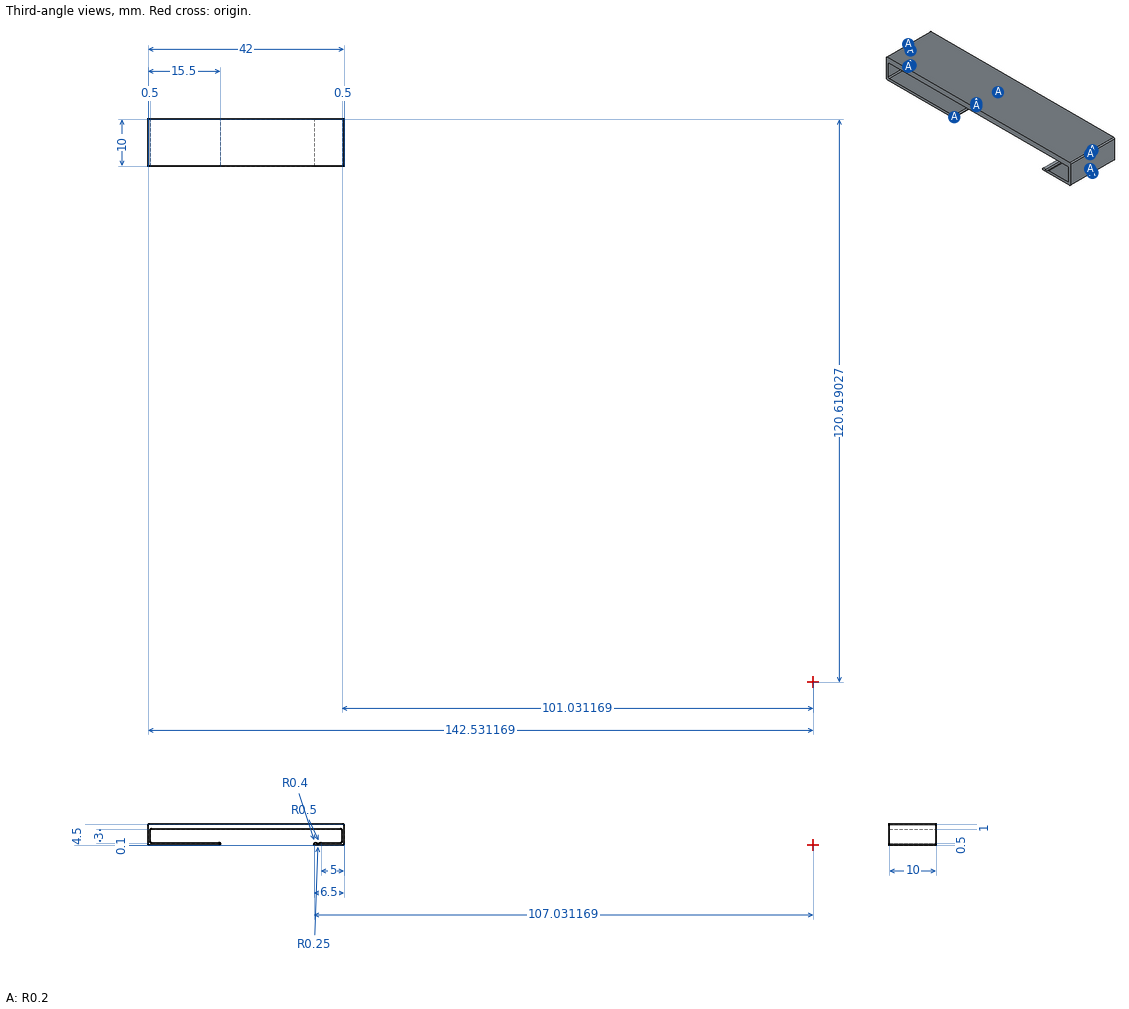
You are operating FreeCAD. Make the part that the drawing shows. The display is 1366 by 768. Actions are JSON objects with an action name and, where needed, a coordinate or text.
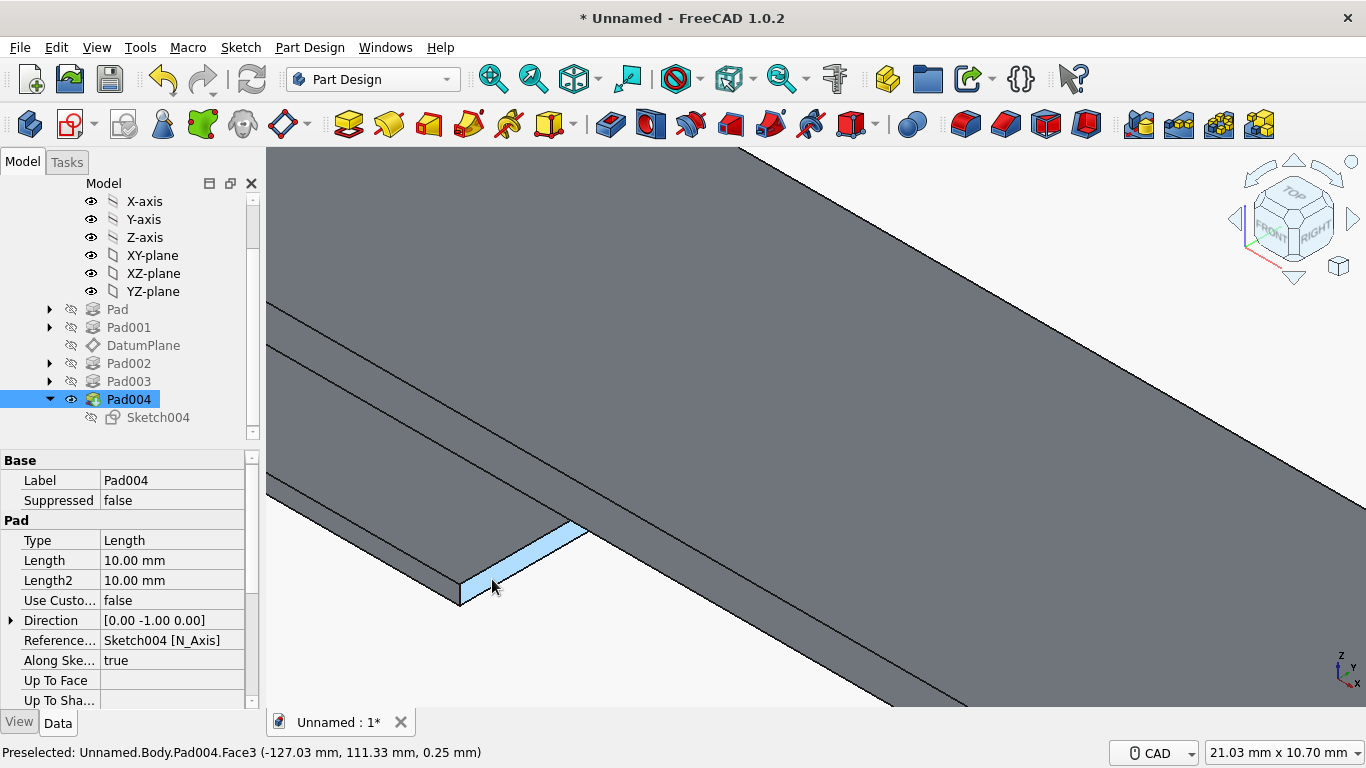
{"action": "left_click", "coordinate": [494, 80]}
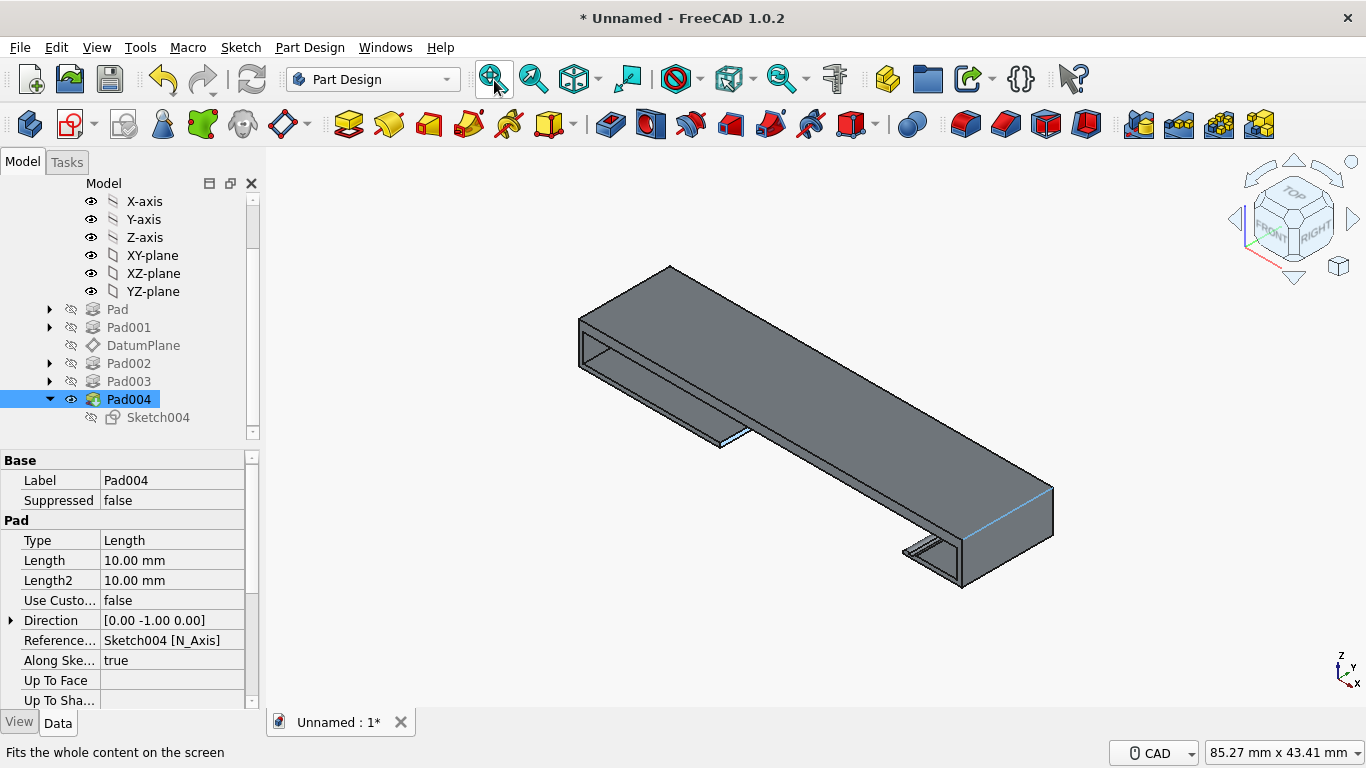
{"action": "key", "text": "2"}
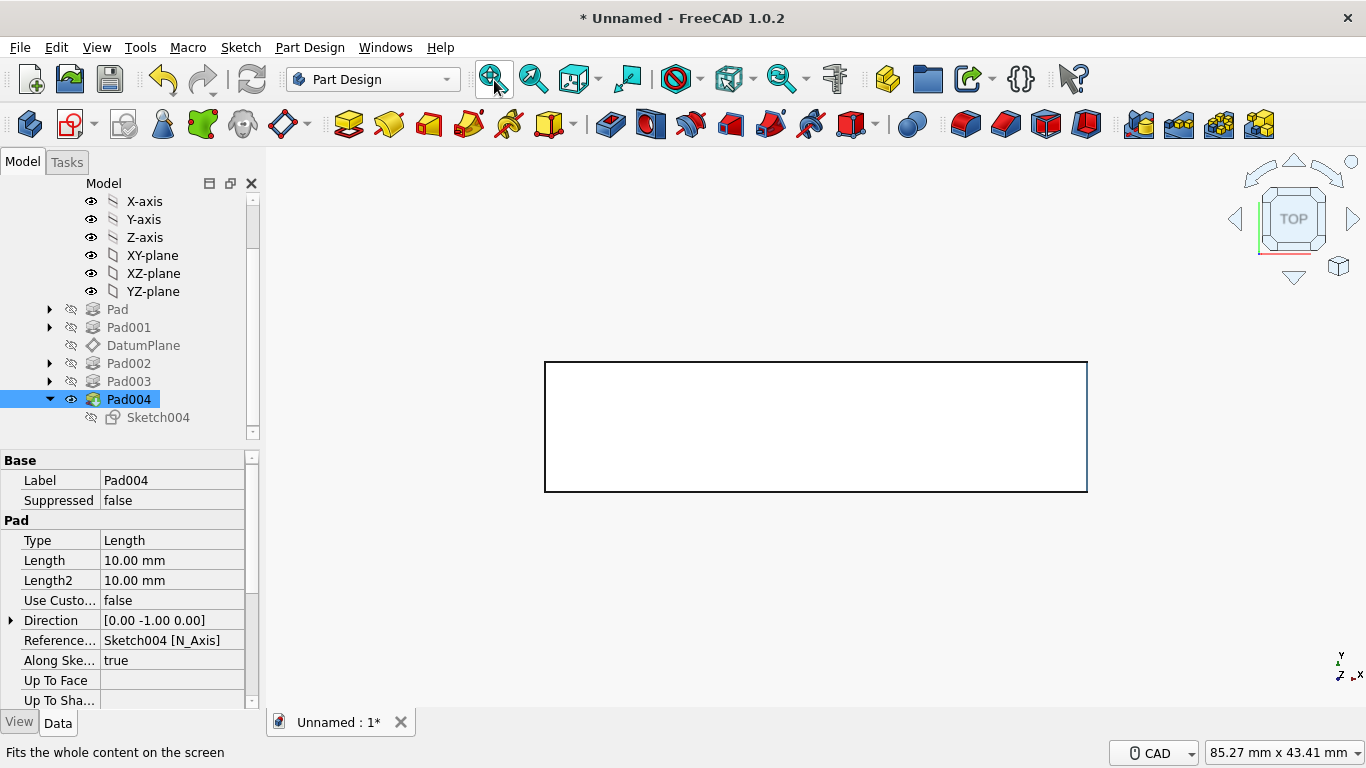
{"action": "left_click", "coordinate": [545, 426], "text": "ctrl"}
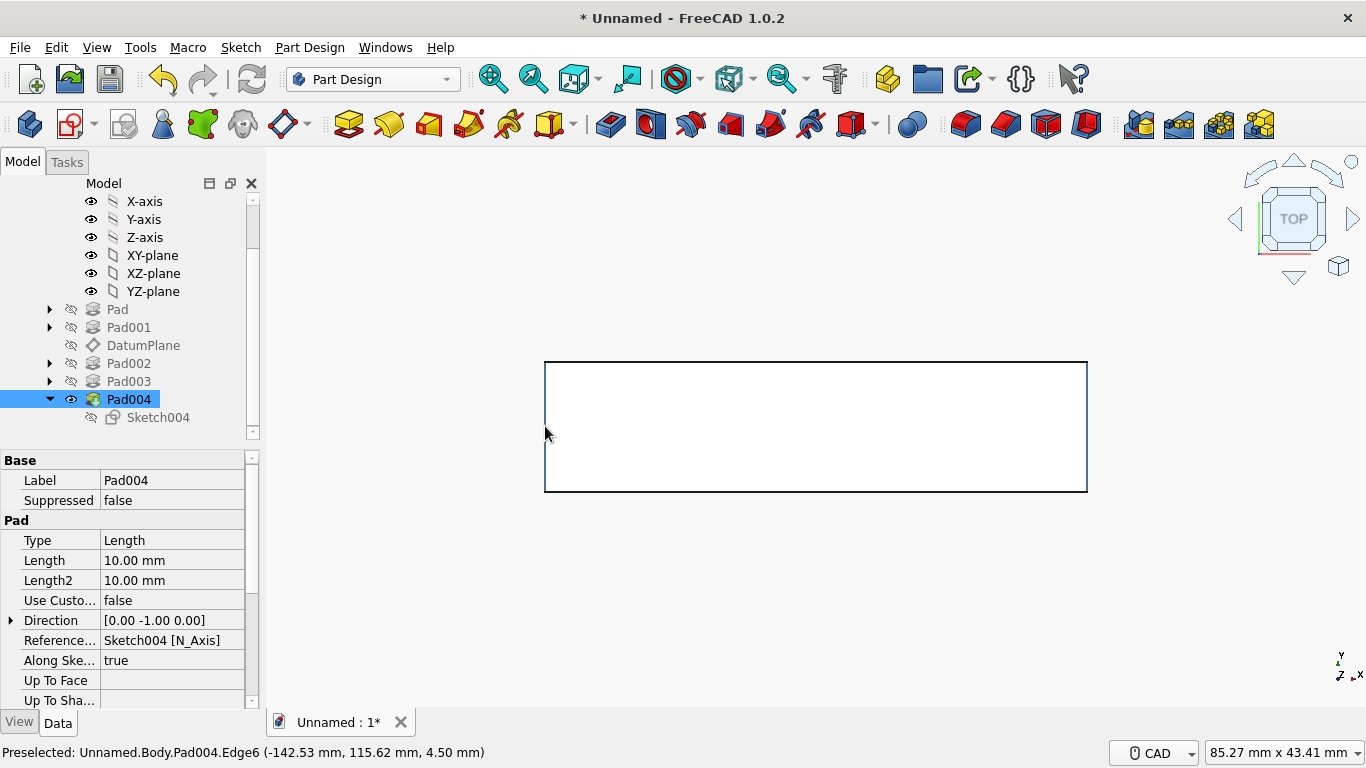
{"action": "key", "text": "0"}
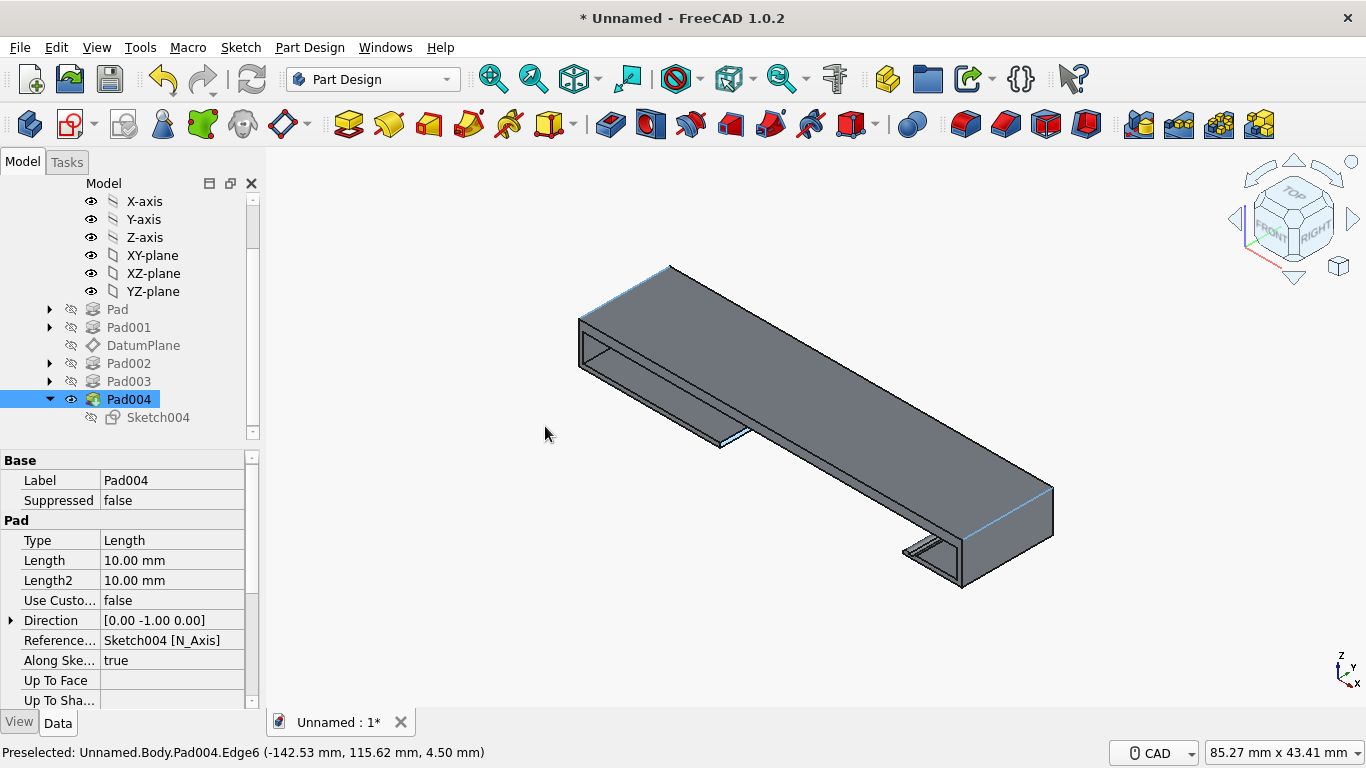
{"action": "key", "text": "1"}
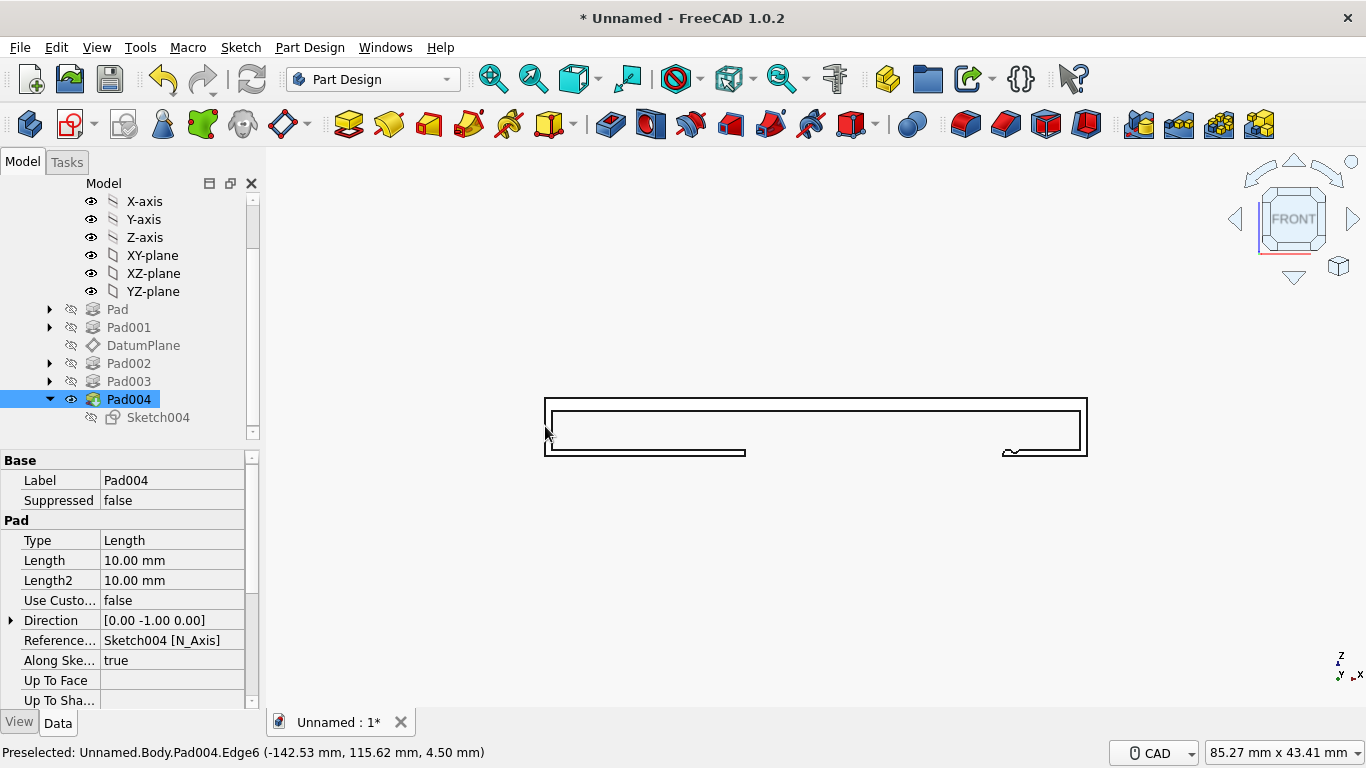
{"action": "key", "text": "3"}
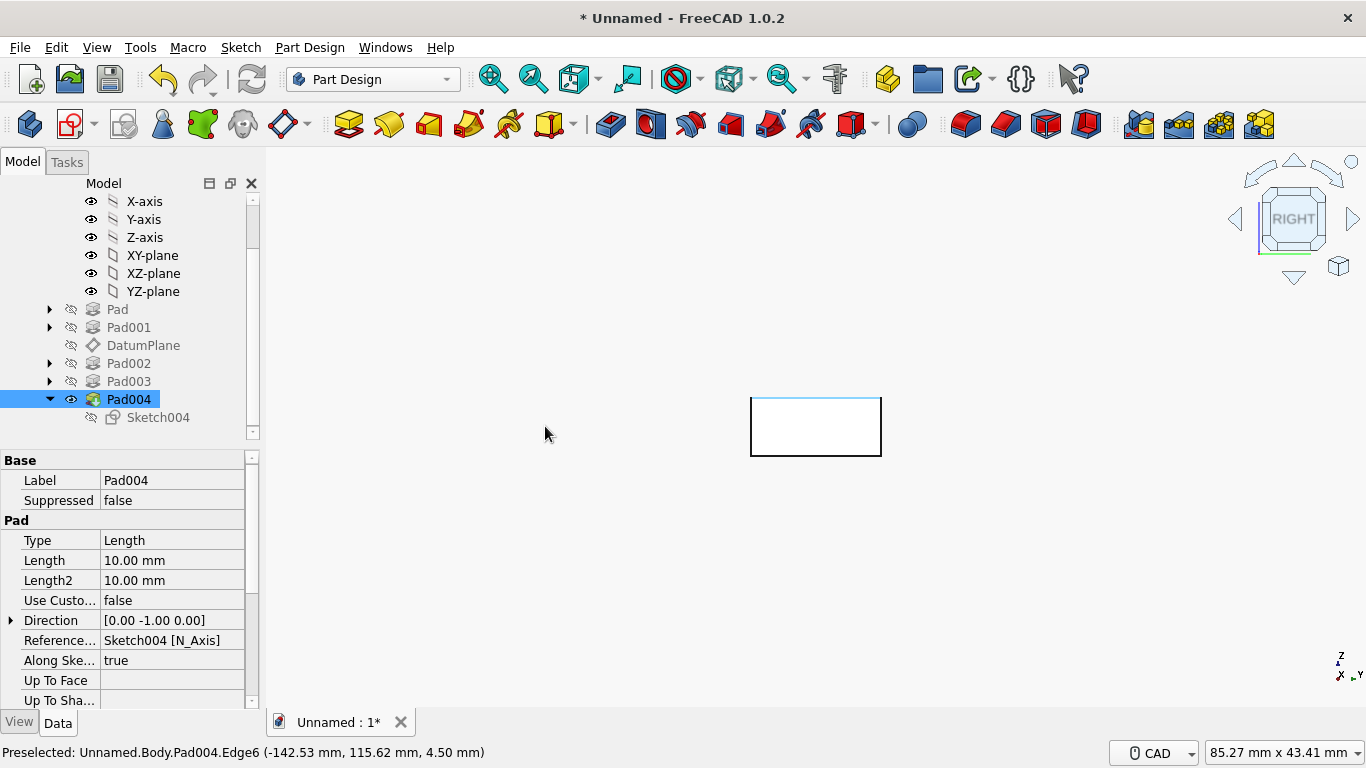
{"action": "left_click", "coordinate": [494, 80]}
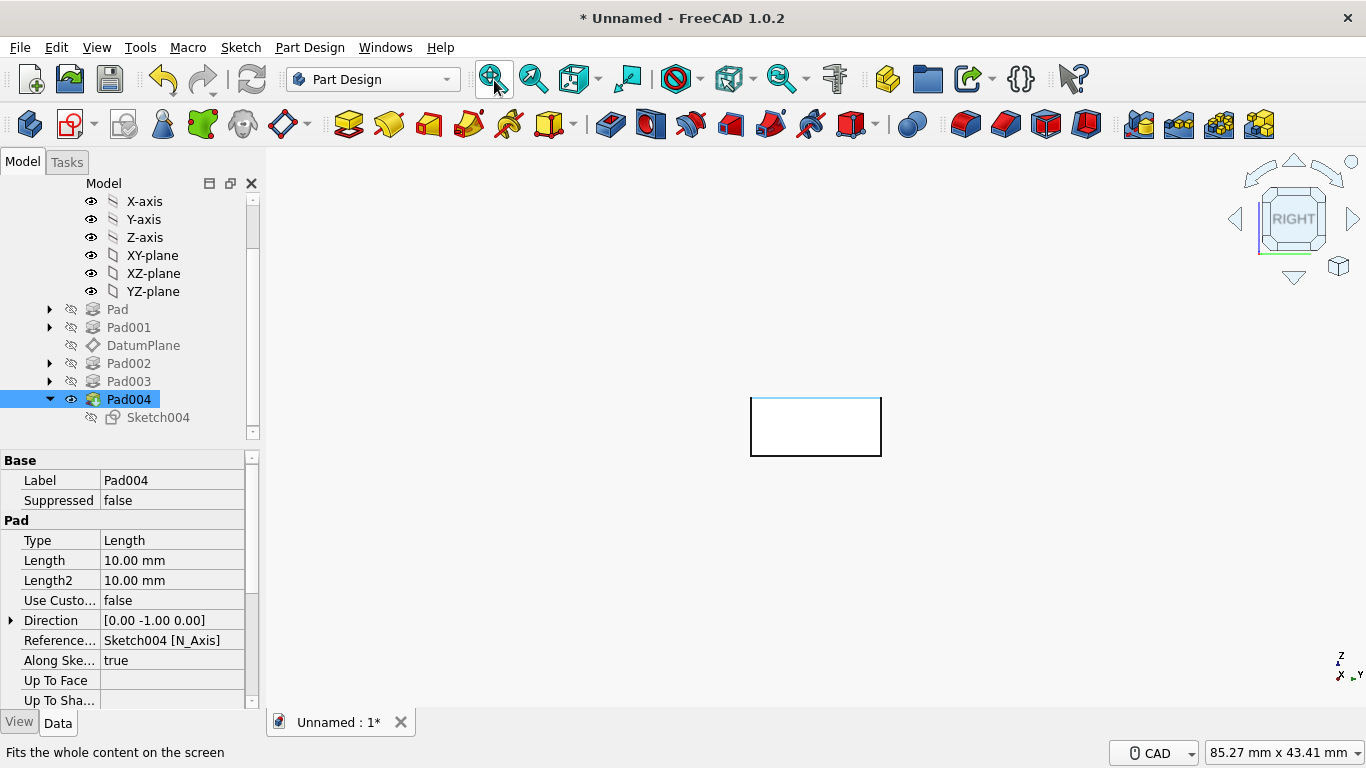
{"action": "left_click", "coordinate": [816, 455], "text": "ctrl"}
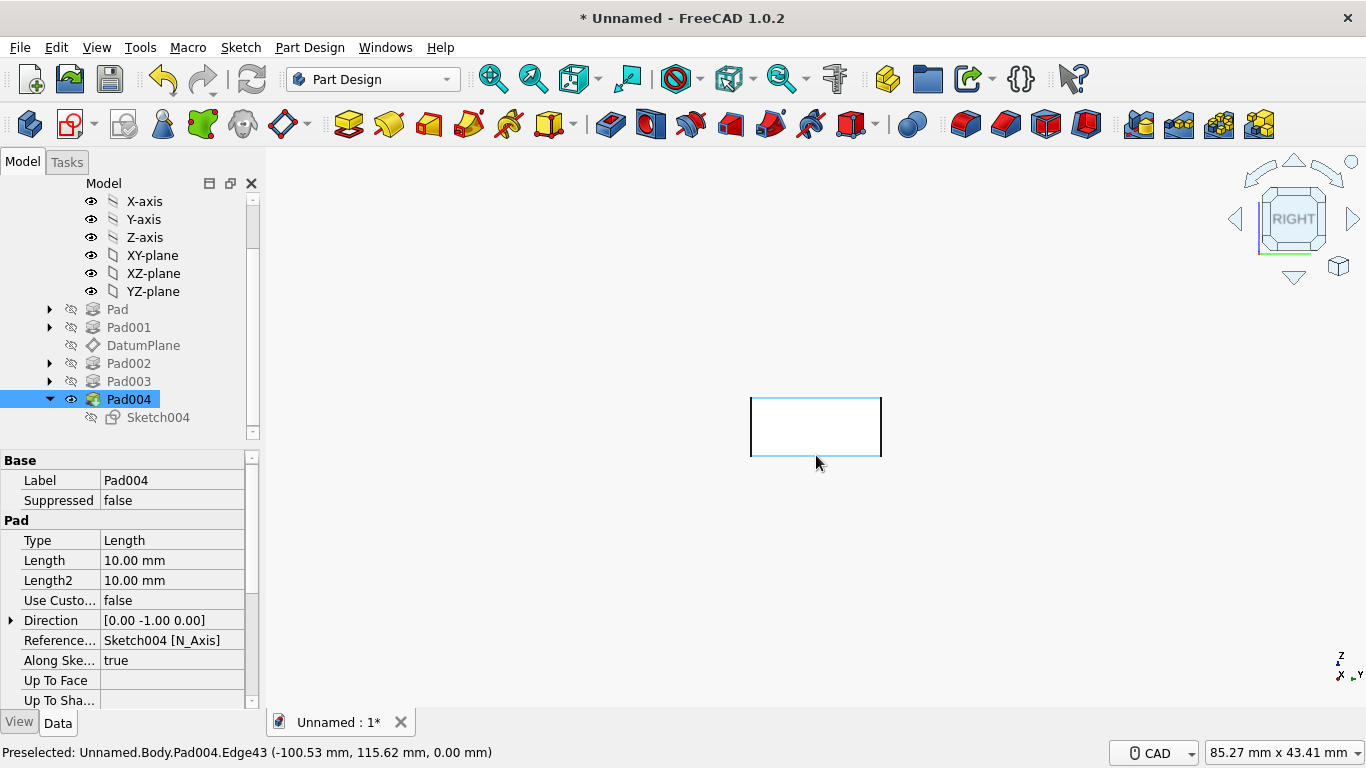
{"action": "key", "text": "5"}